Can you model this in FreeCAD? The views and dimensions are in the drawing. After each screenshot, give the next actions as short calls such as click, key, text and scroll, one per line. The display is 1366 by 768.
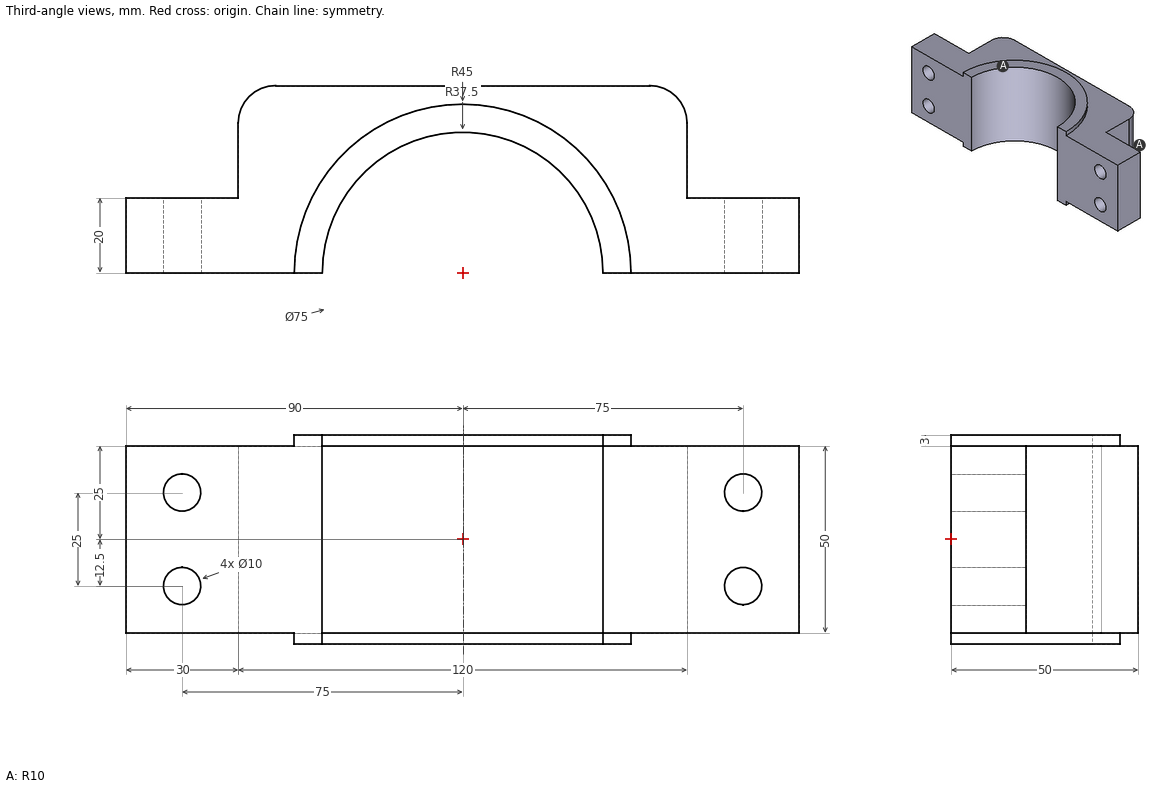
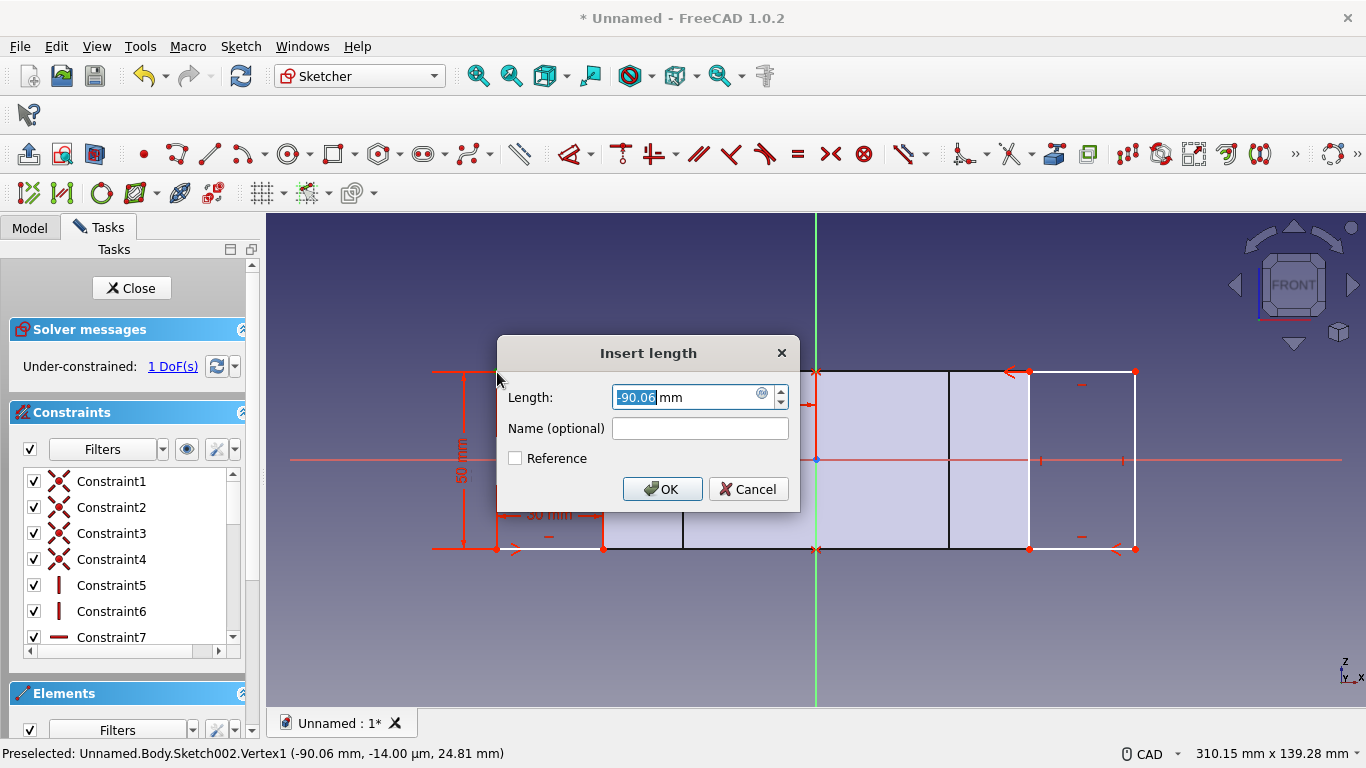
text(-90)
key(Return)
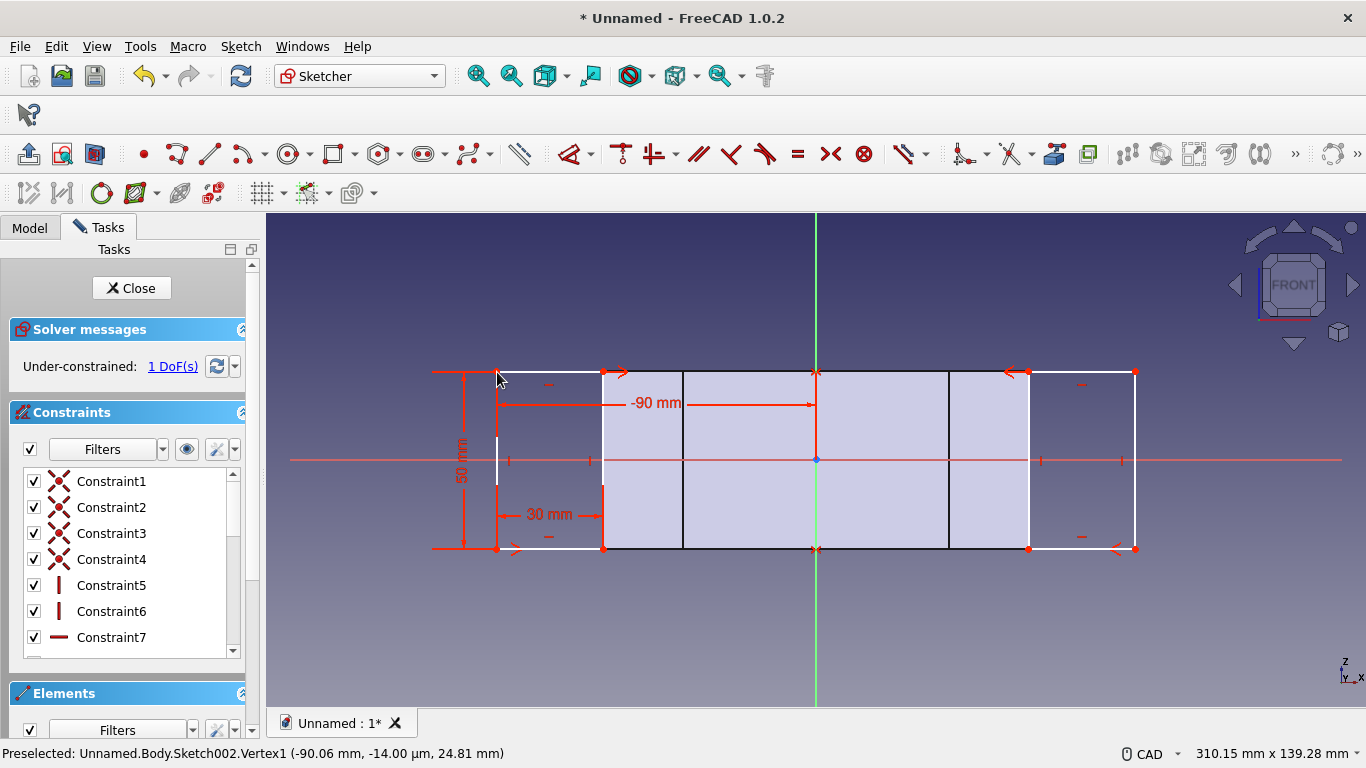
click(497, 372)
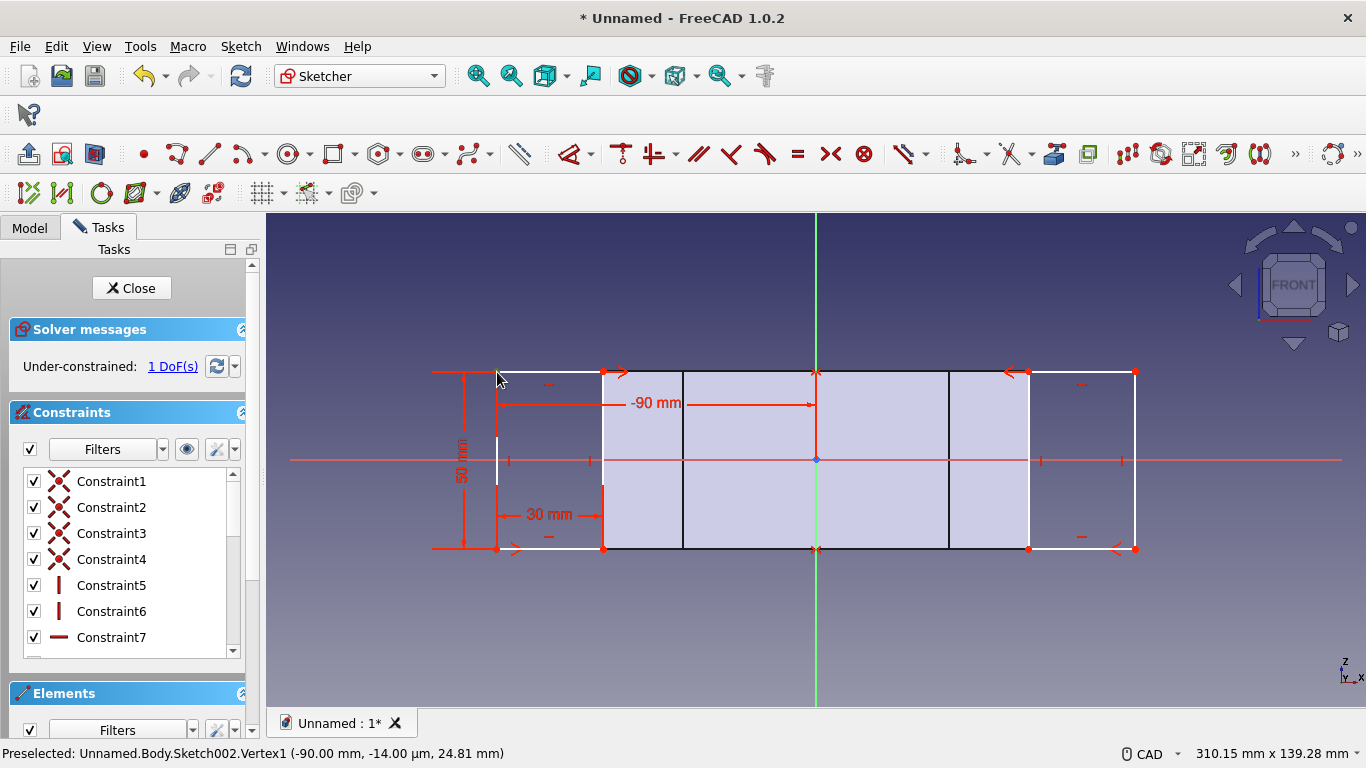
key(i)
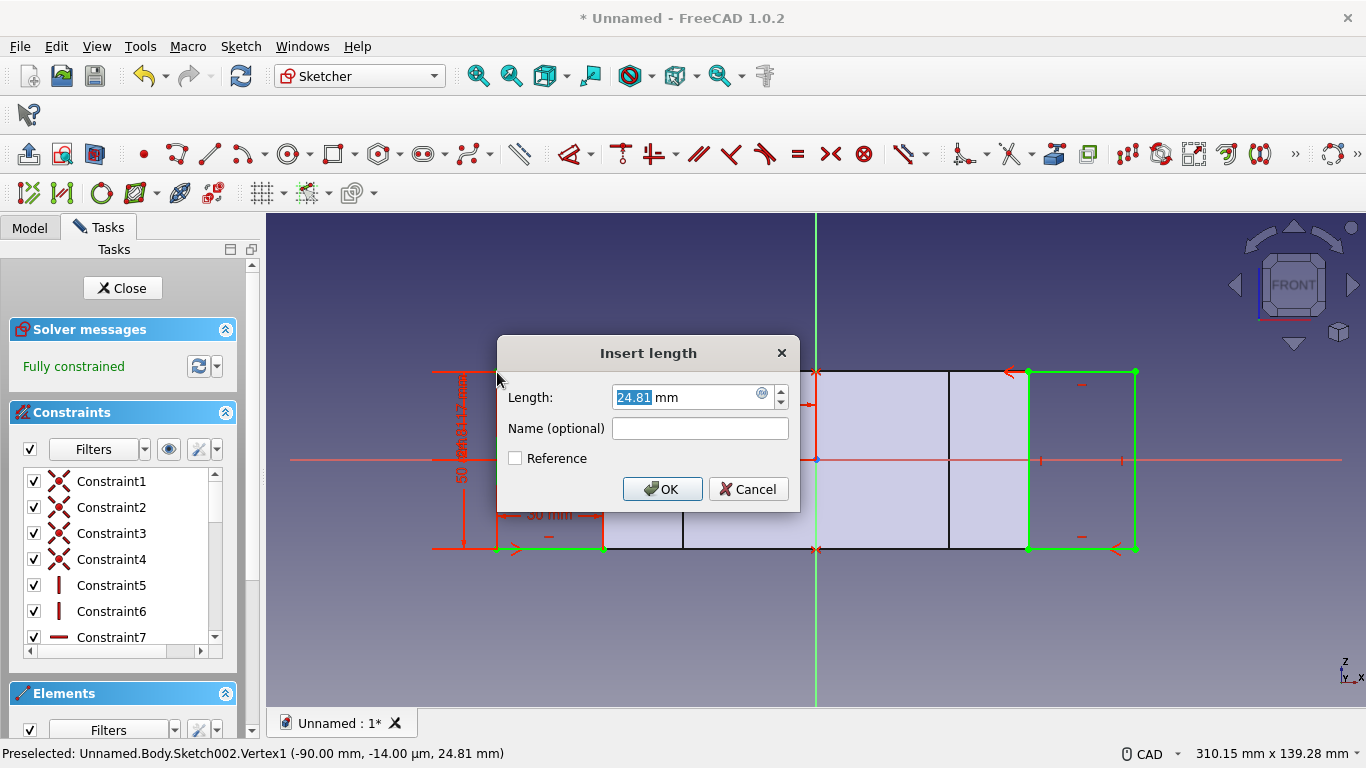
text(25)
key(Return)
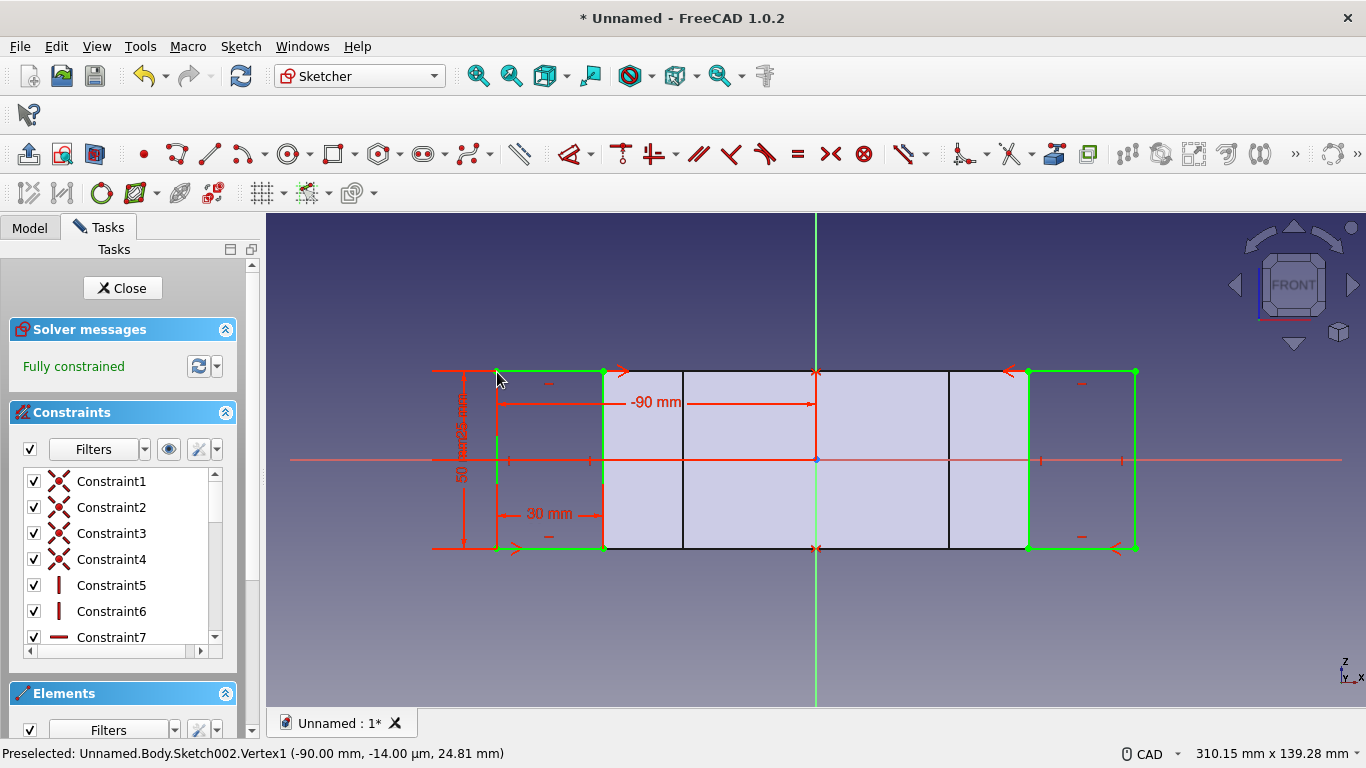
click(123, 288)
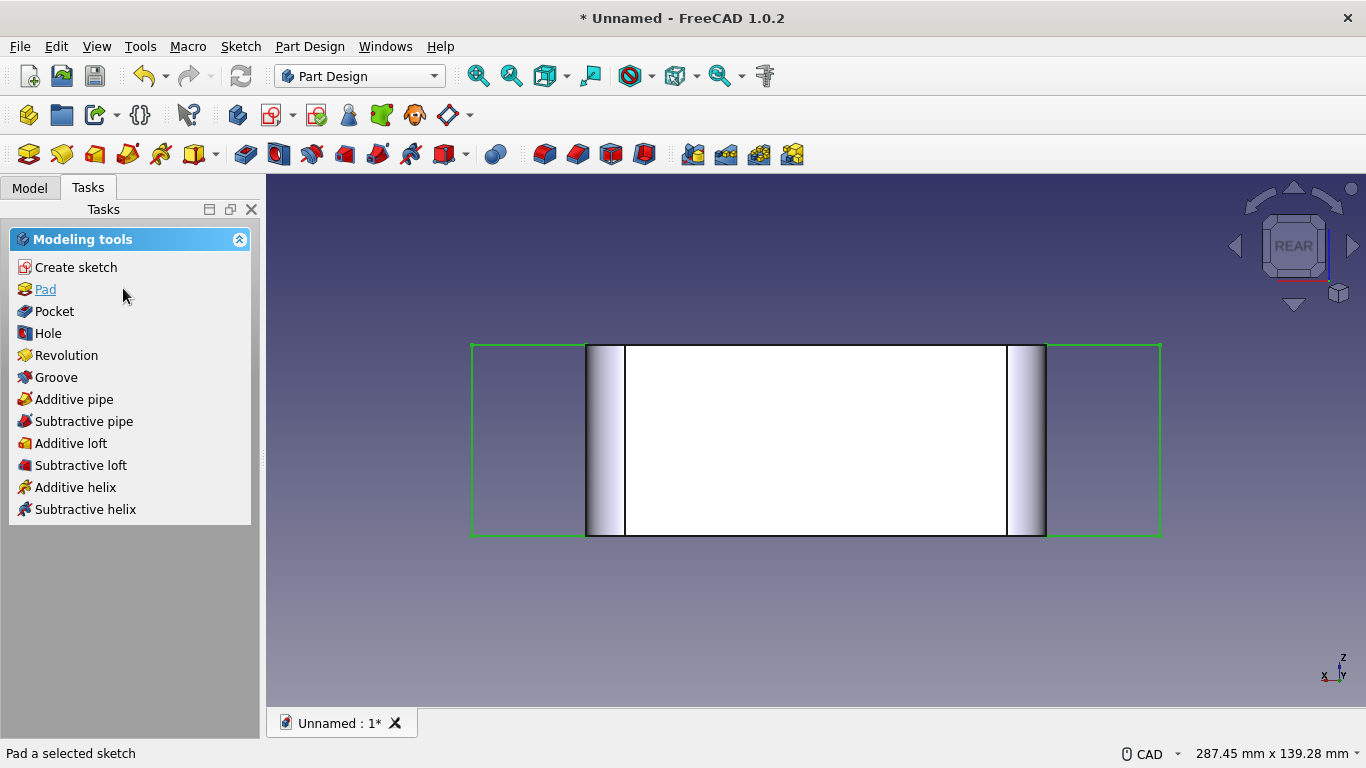
click(29, 154)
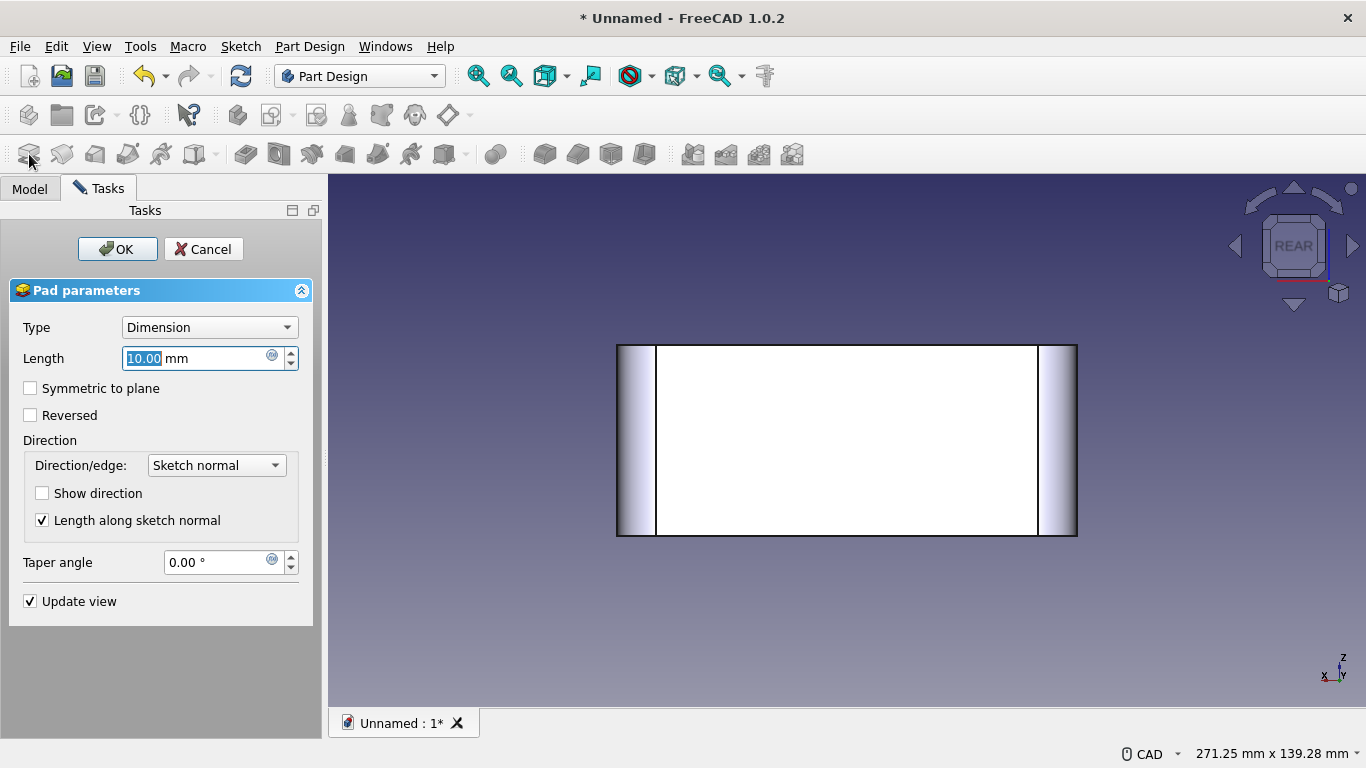
text(20)
key(Tab)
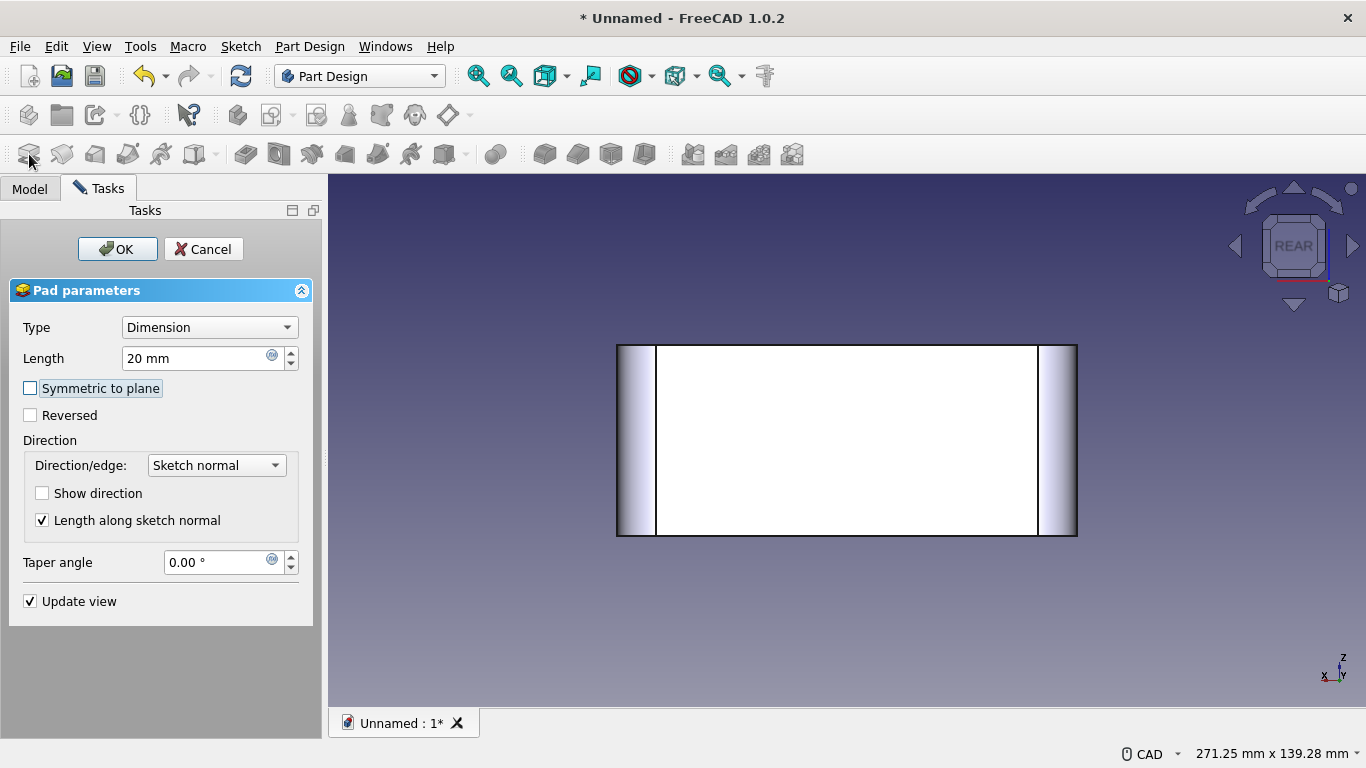
click(31, 415)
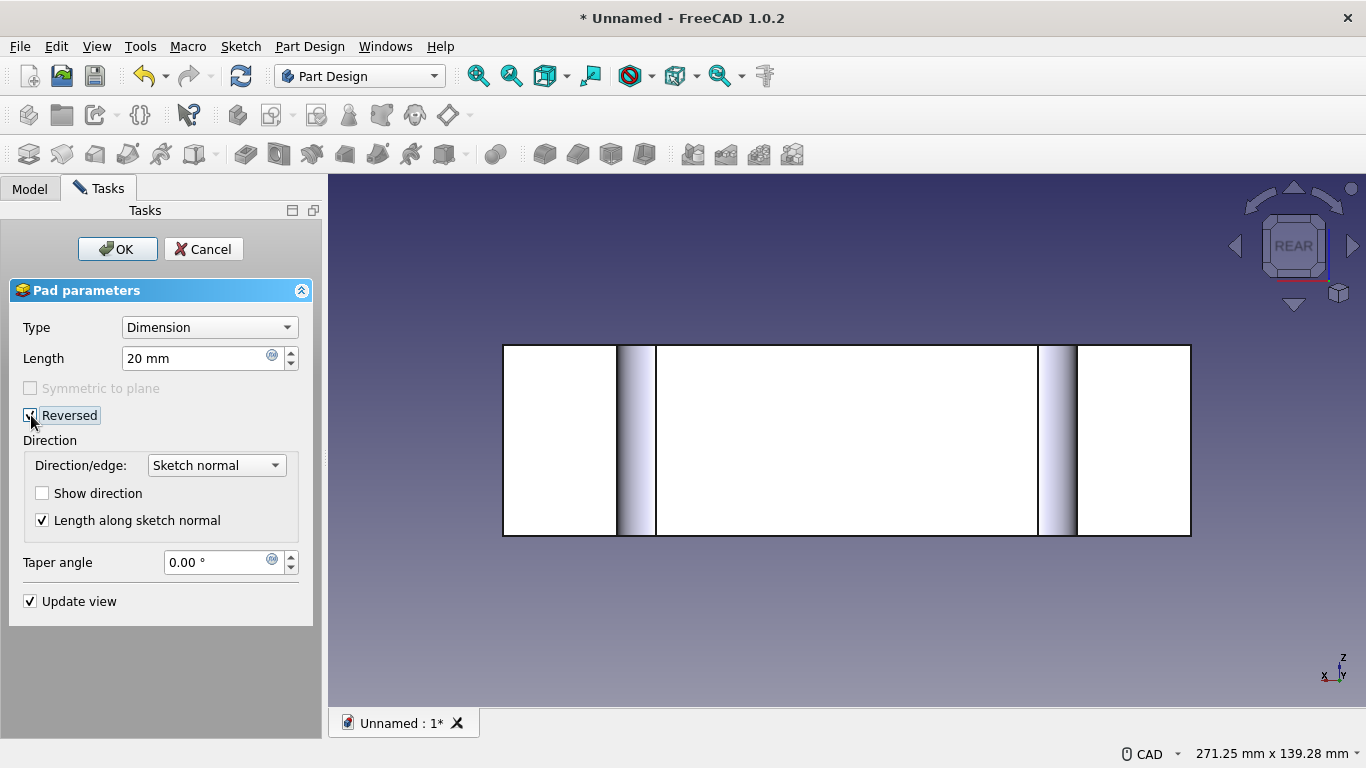
click(118, 249)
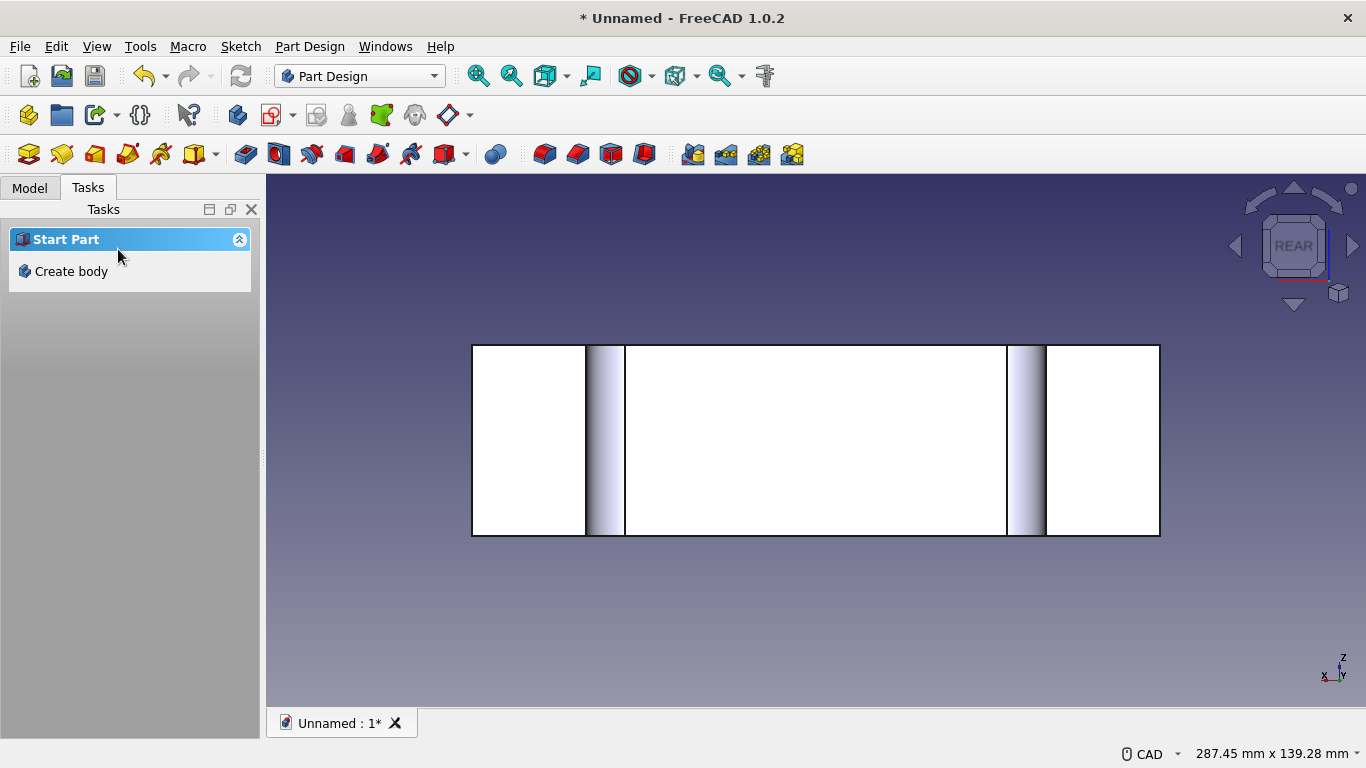
click(30, 188)